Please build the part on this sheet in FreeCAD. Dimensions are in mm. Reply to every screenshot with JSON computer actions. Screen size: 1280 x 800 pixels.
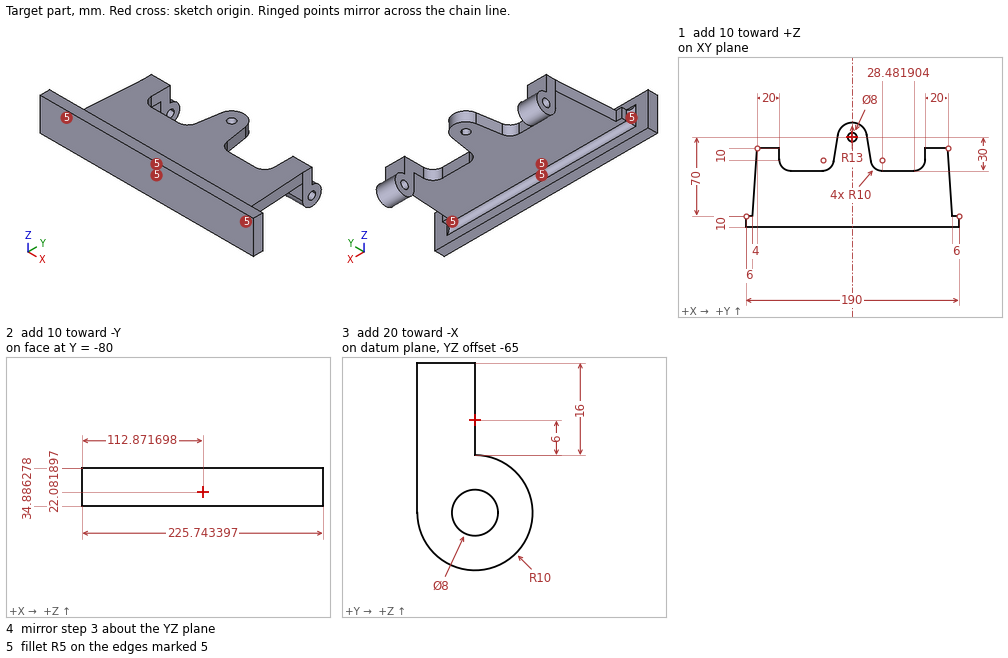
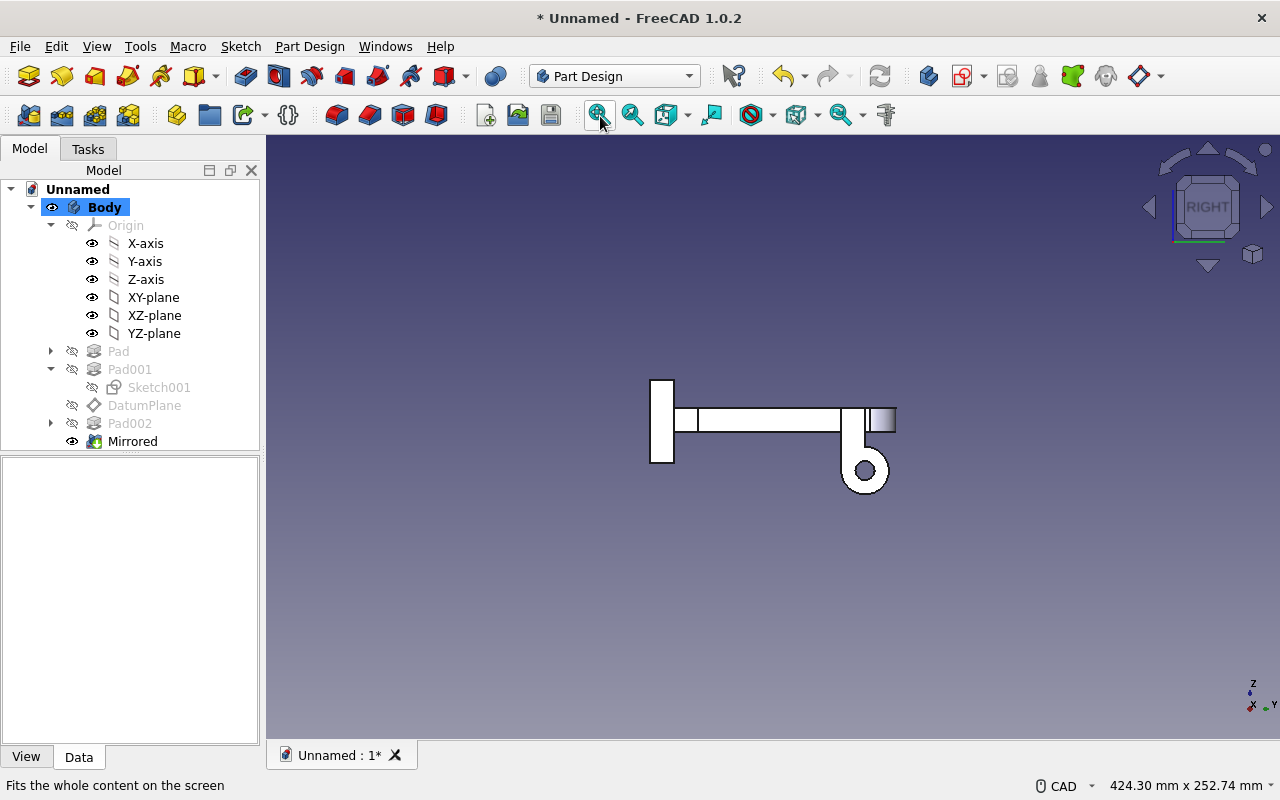
{"action": "key", "text": "5"}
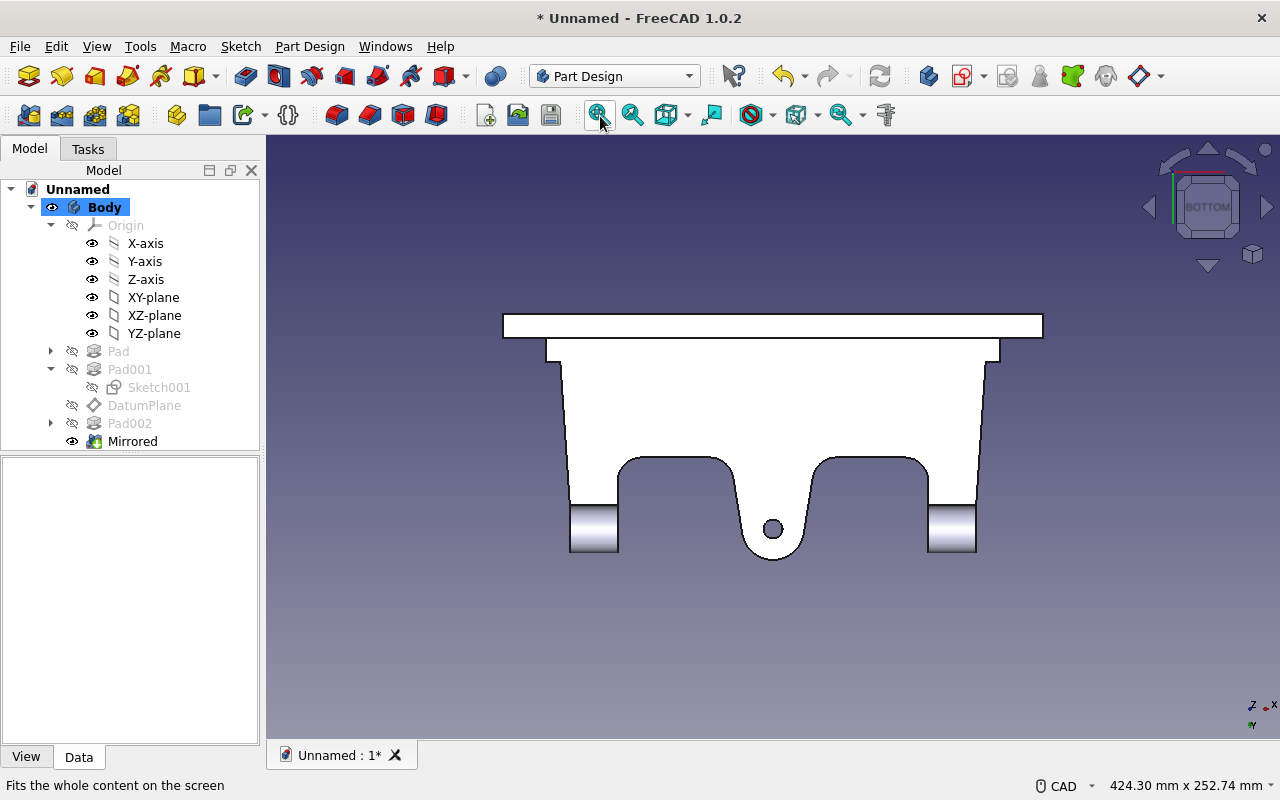
{"action": "key", "text": "4"}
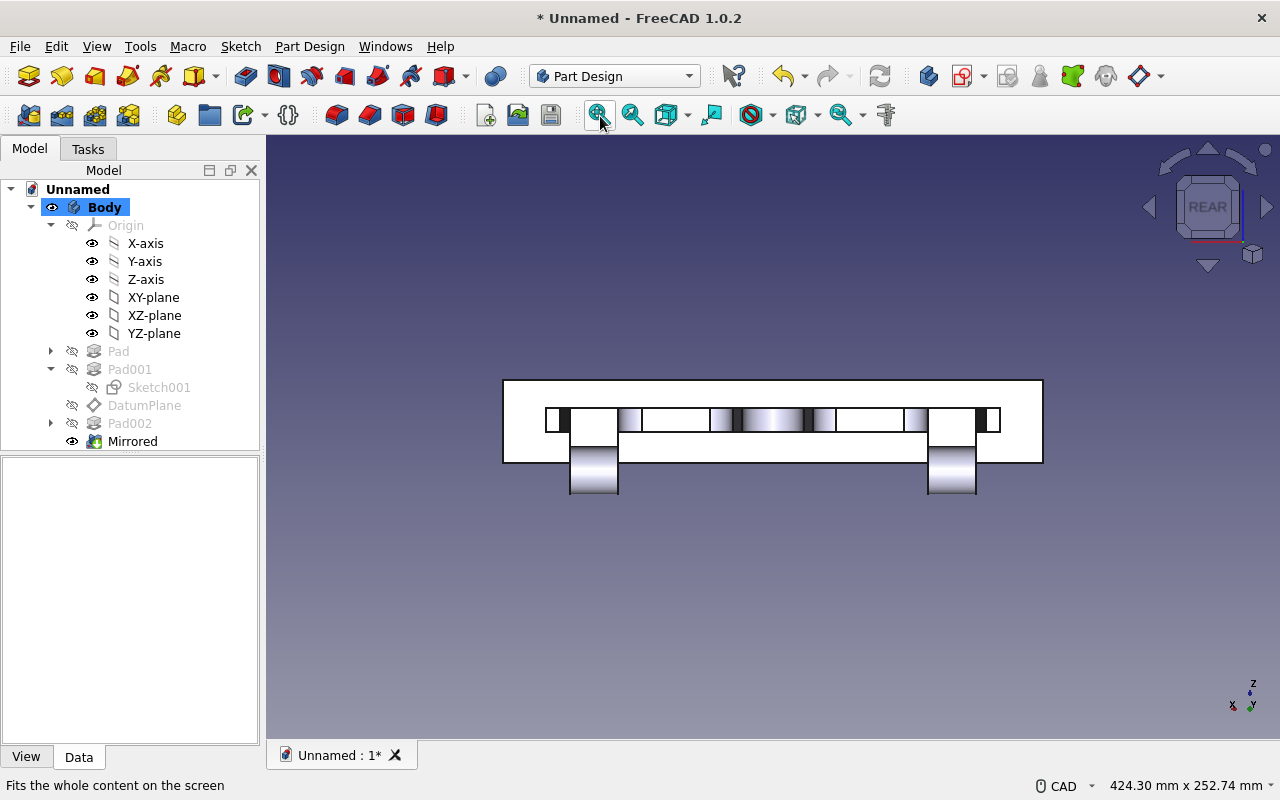
{"action": "key", "text": "6"}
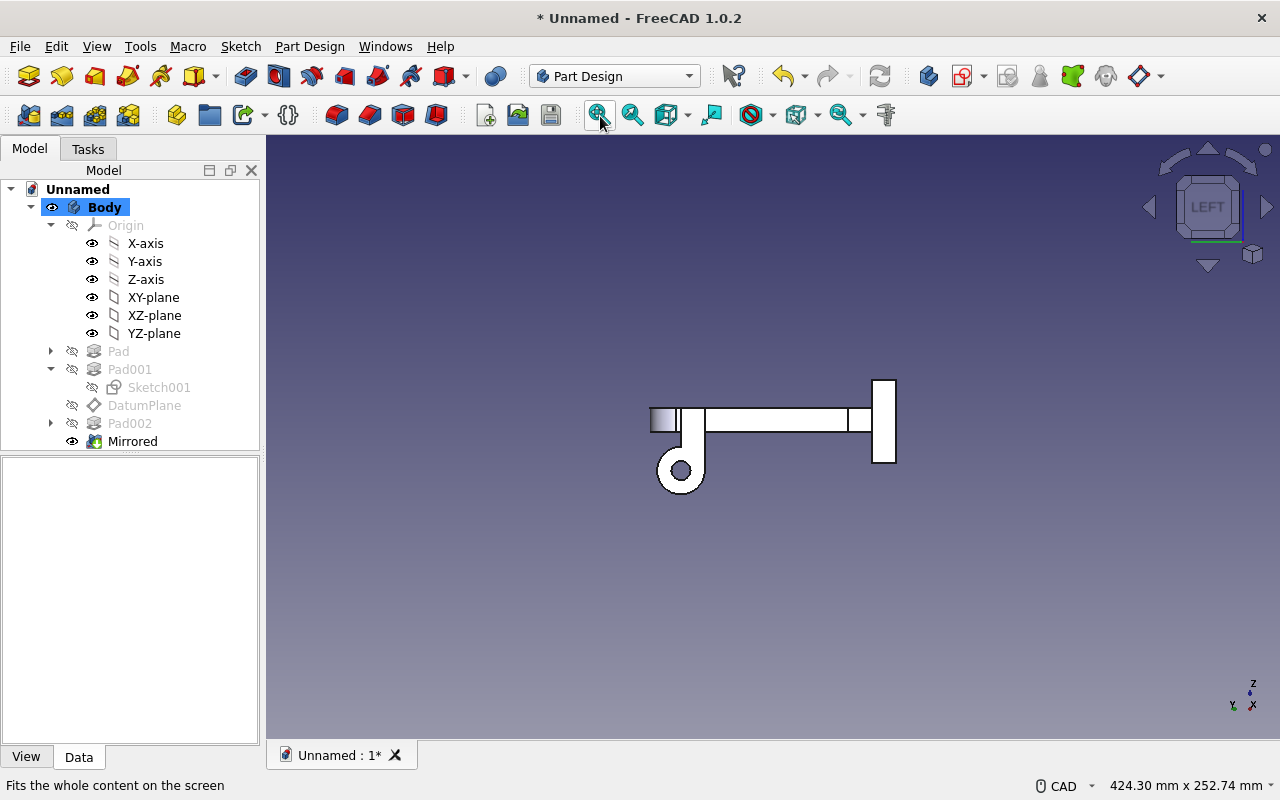
{"action": "key", "text": "v f"}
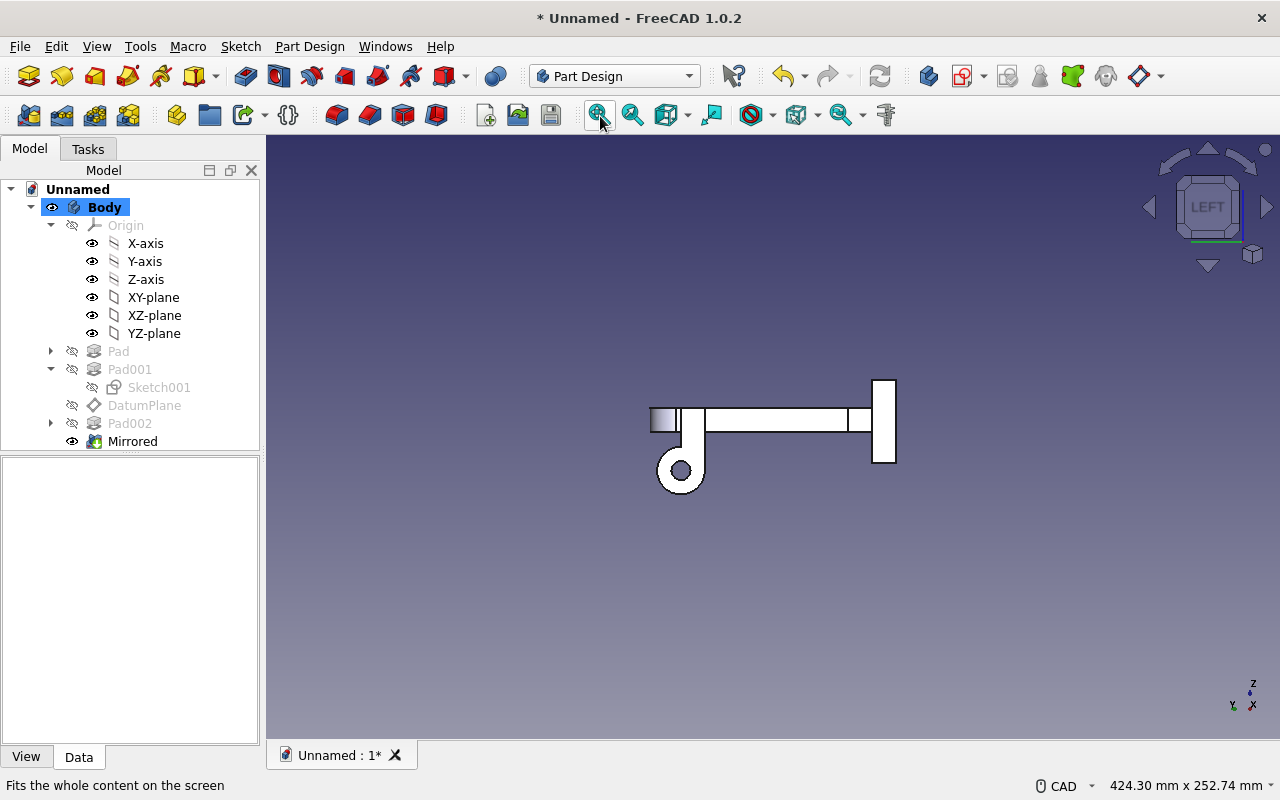
{"action": "key", "text": "v 3"}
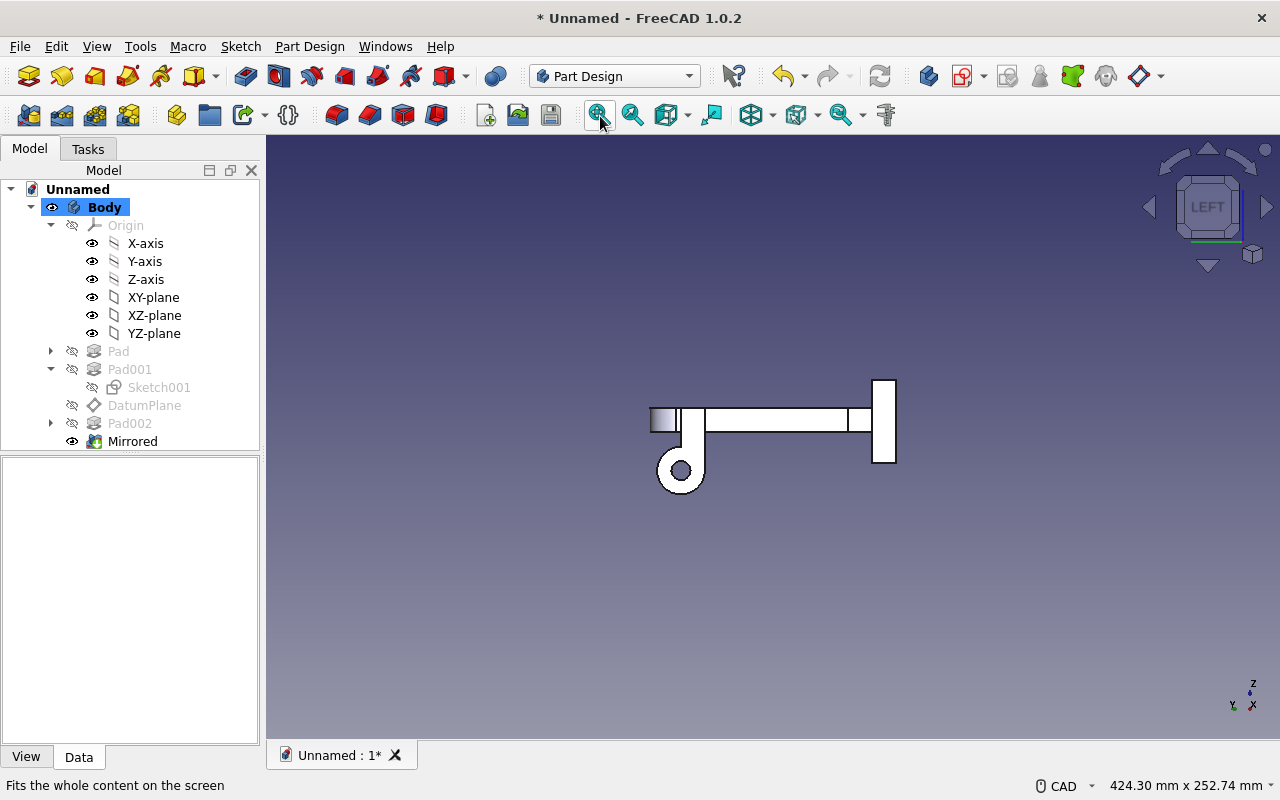
{"action": "key", "text": "0"}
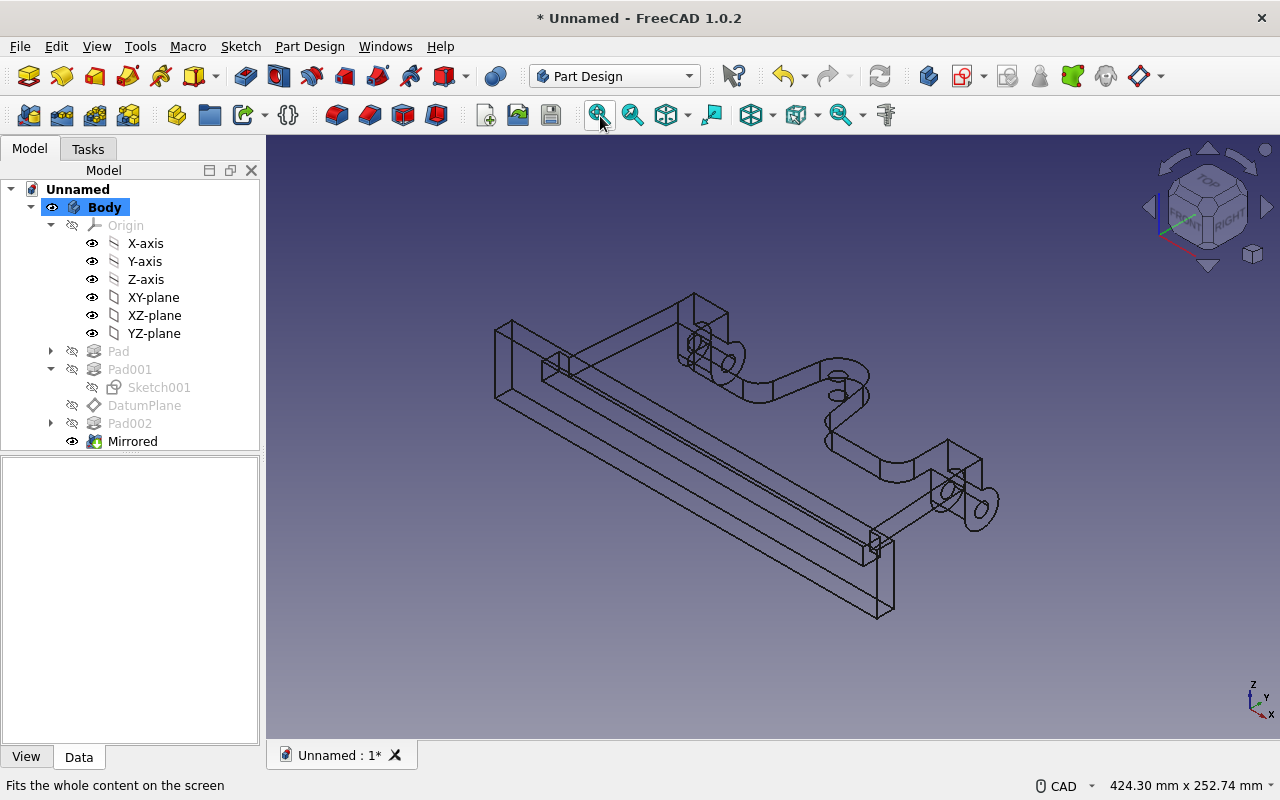
{"action": "left_click", "coordinate": [703, 473]}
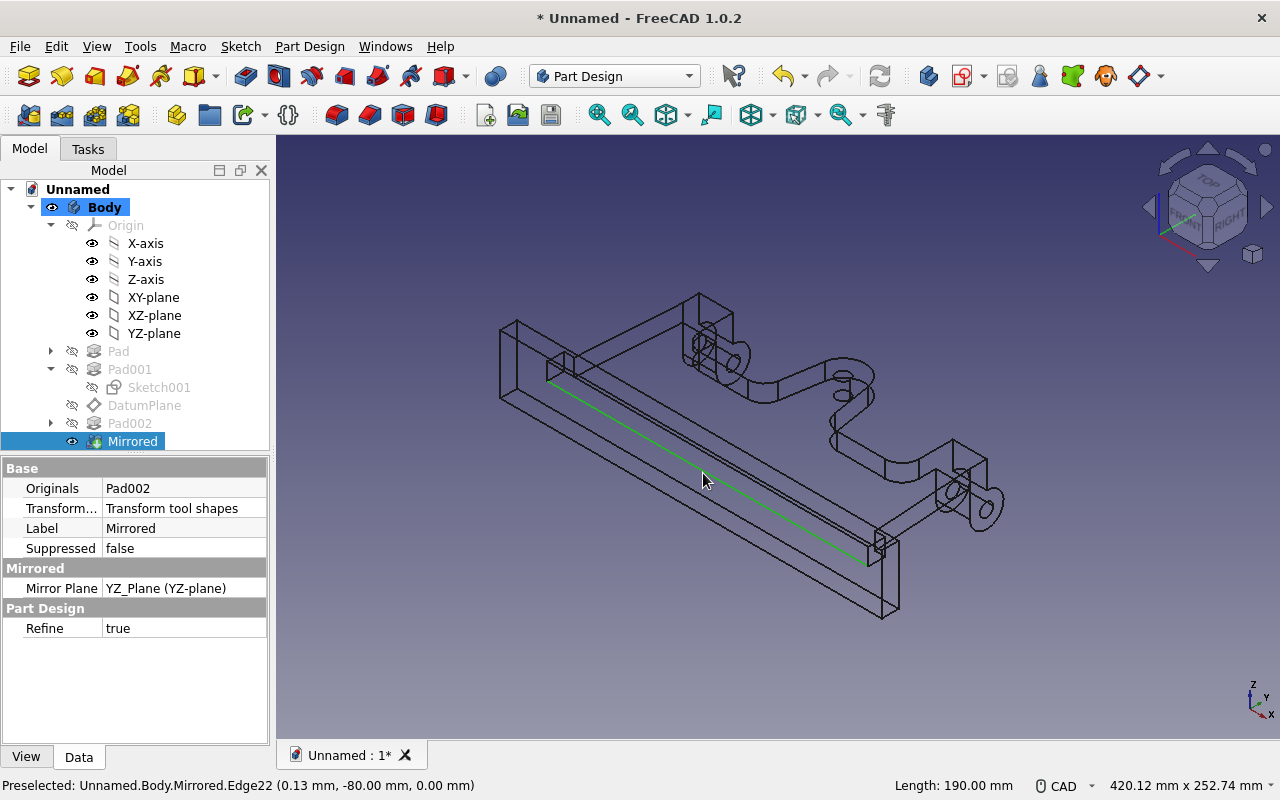
{"action": "left_click", "coordinate": [868, 556], "text": "ctrl"}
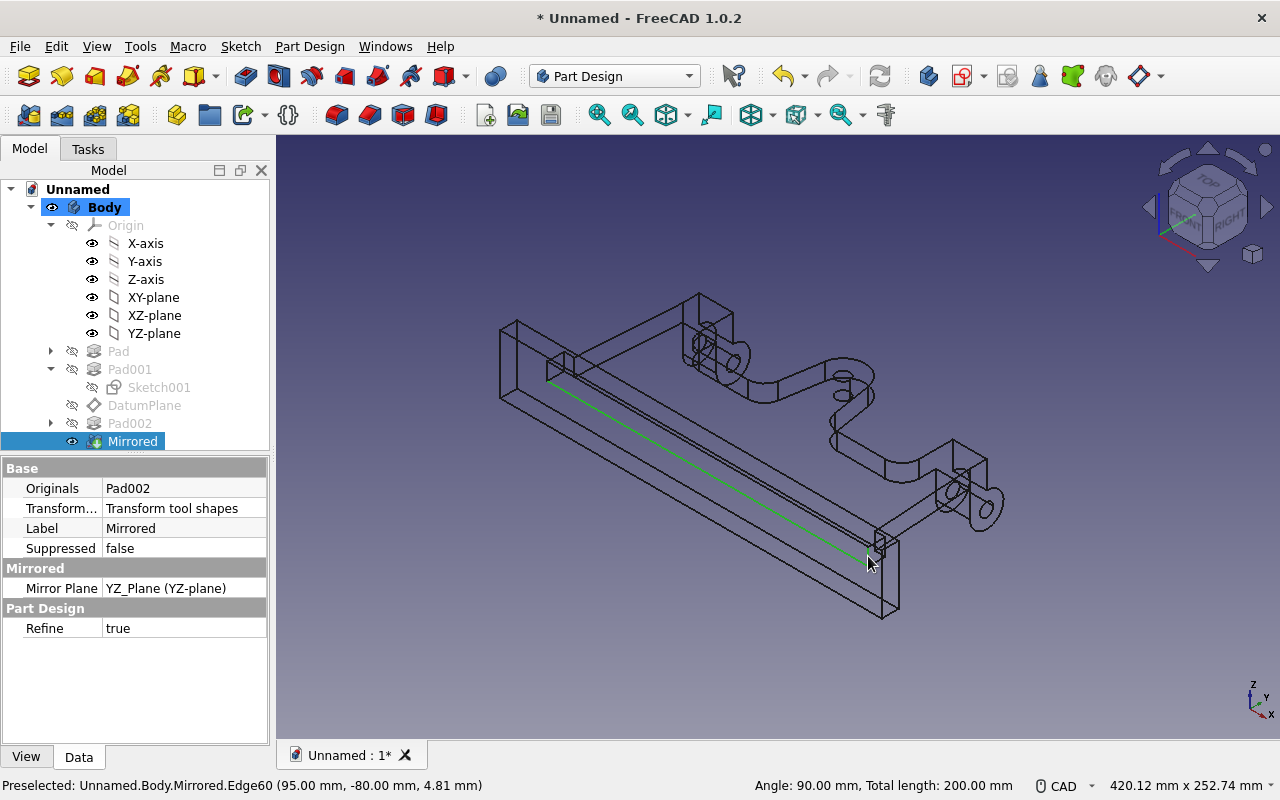
{"action": "left_click", "coordinate": [547, 370], "text": "ctrl"}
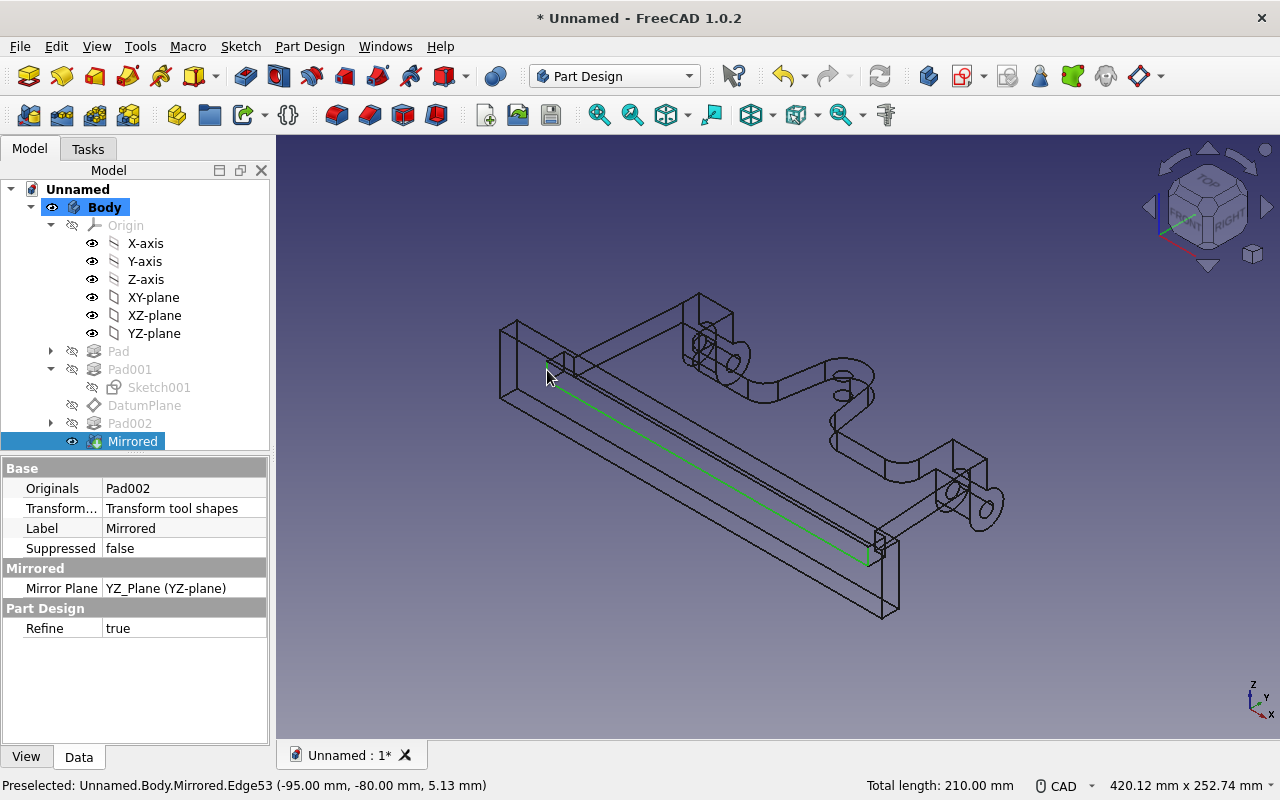
{"action": "scroll", "coordinate": [708, 453], "scroll_direction": "up", "scroll_amount": 6}